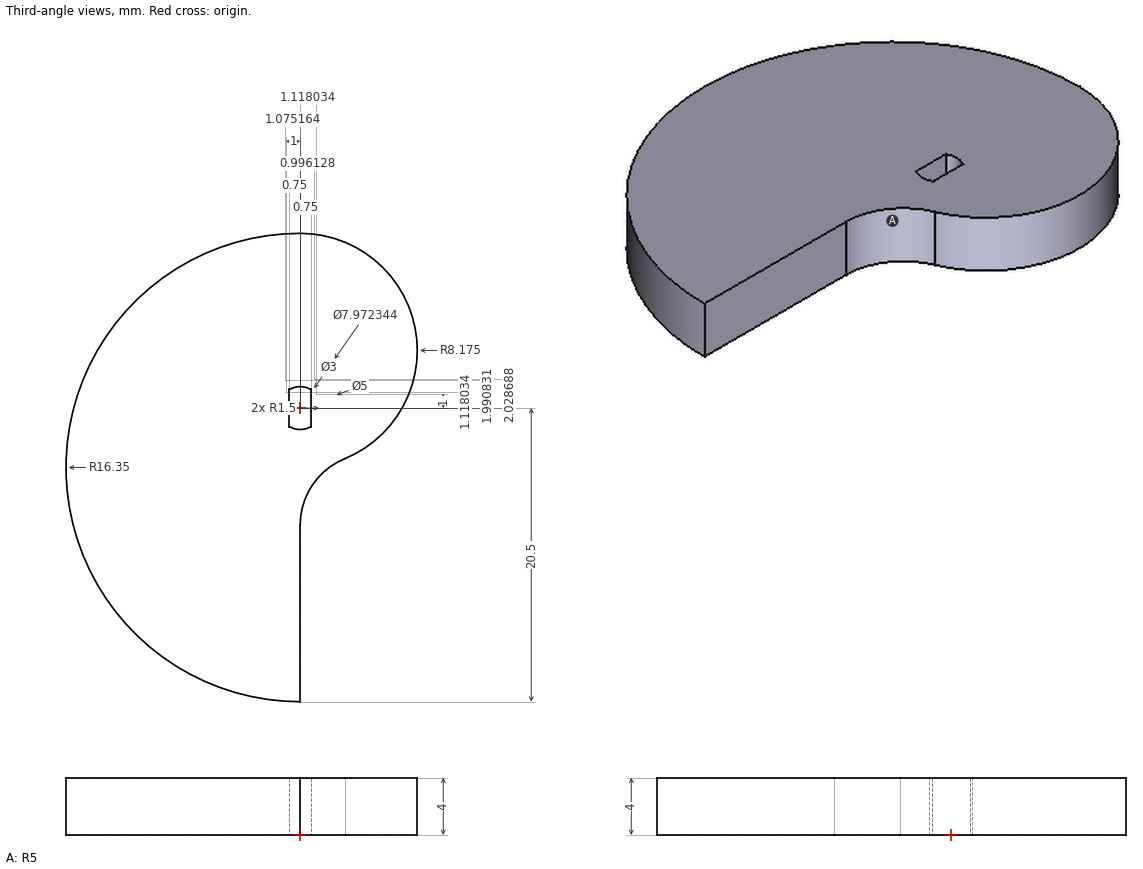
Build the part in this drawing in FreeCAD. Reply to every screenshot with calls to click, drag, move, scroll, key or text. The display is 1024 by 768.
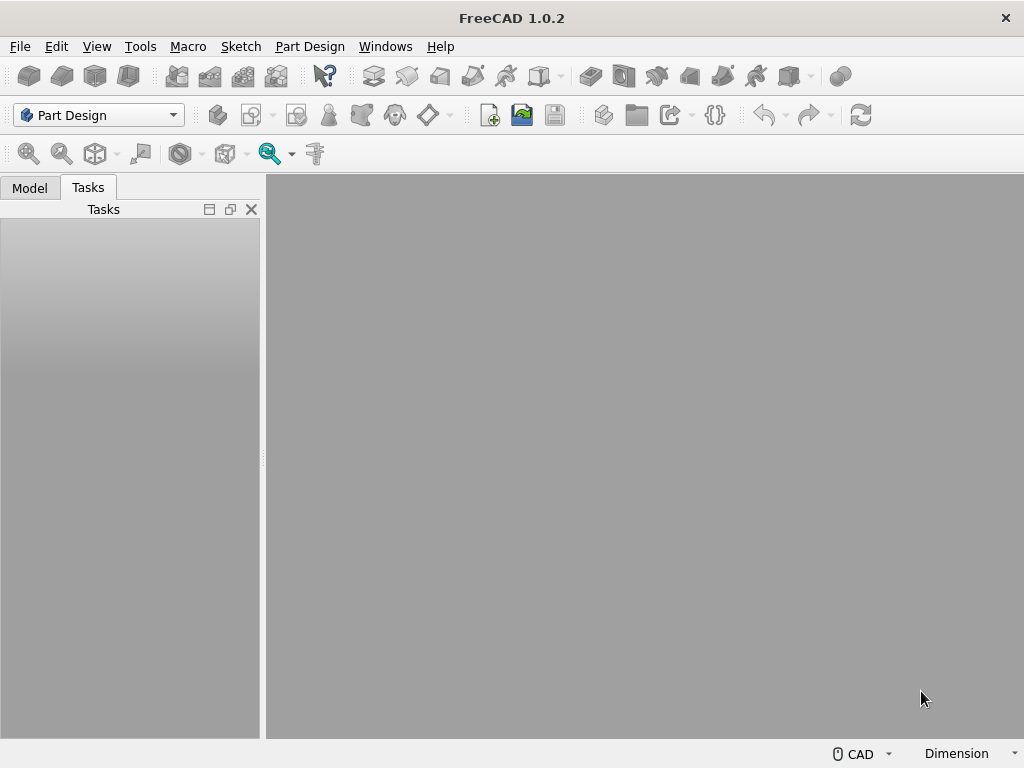
key(ctrl+n)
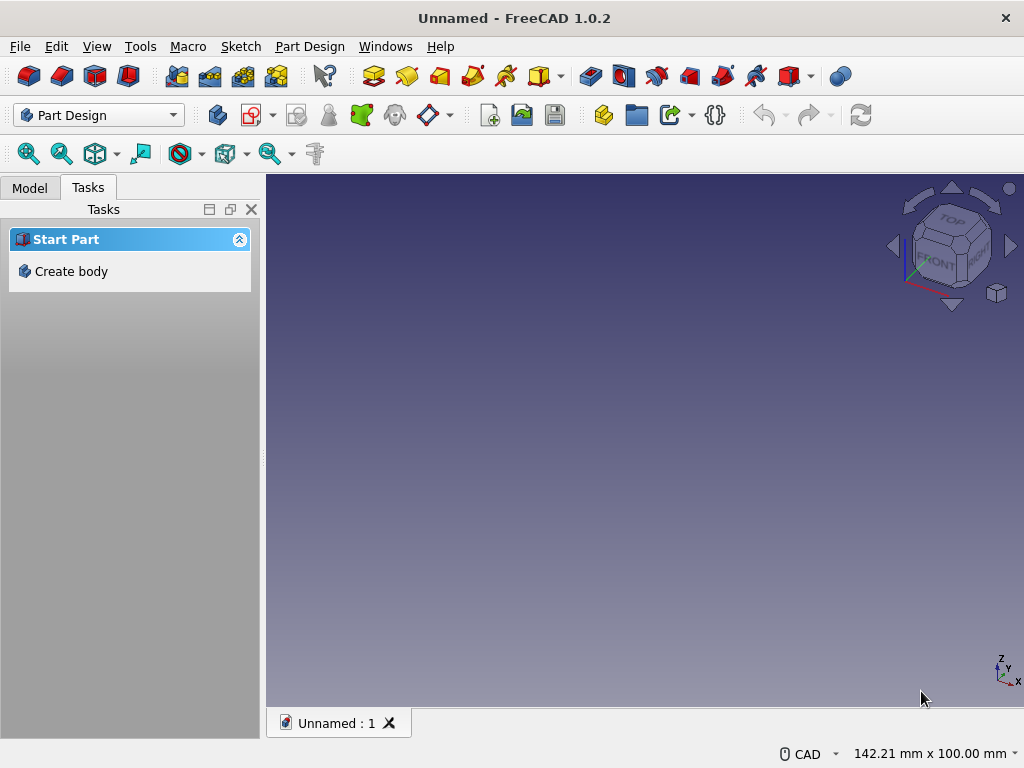
click(250, 116)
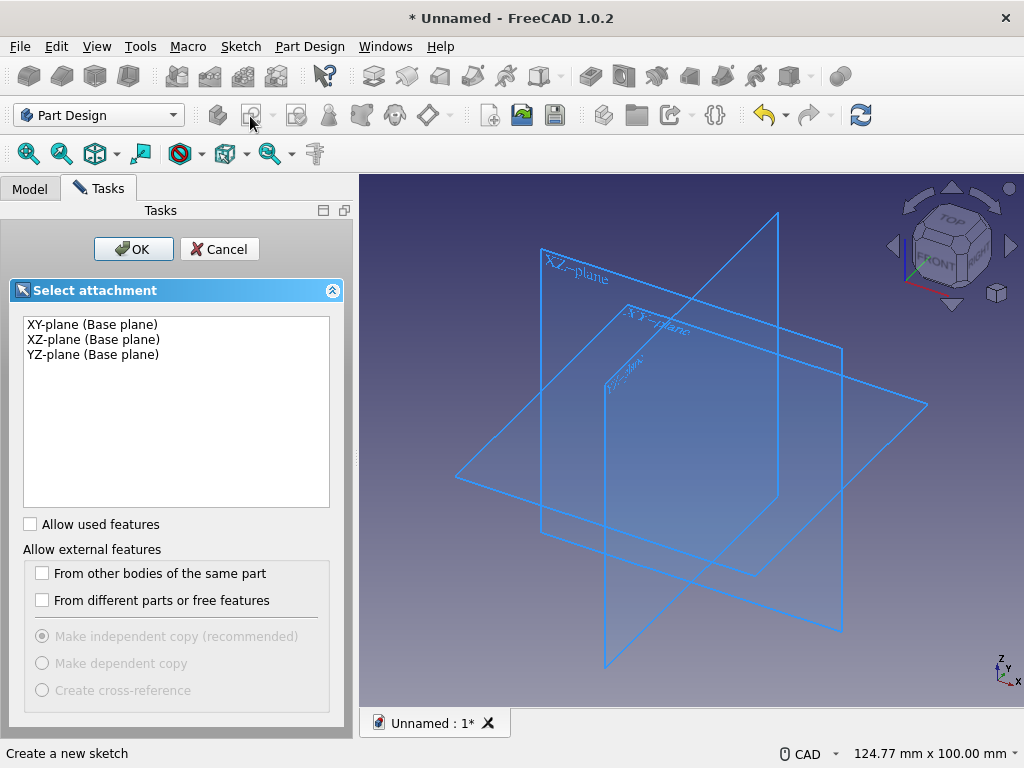
click(84, 324)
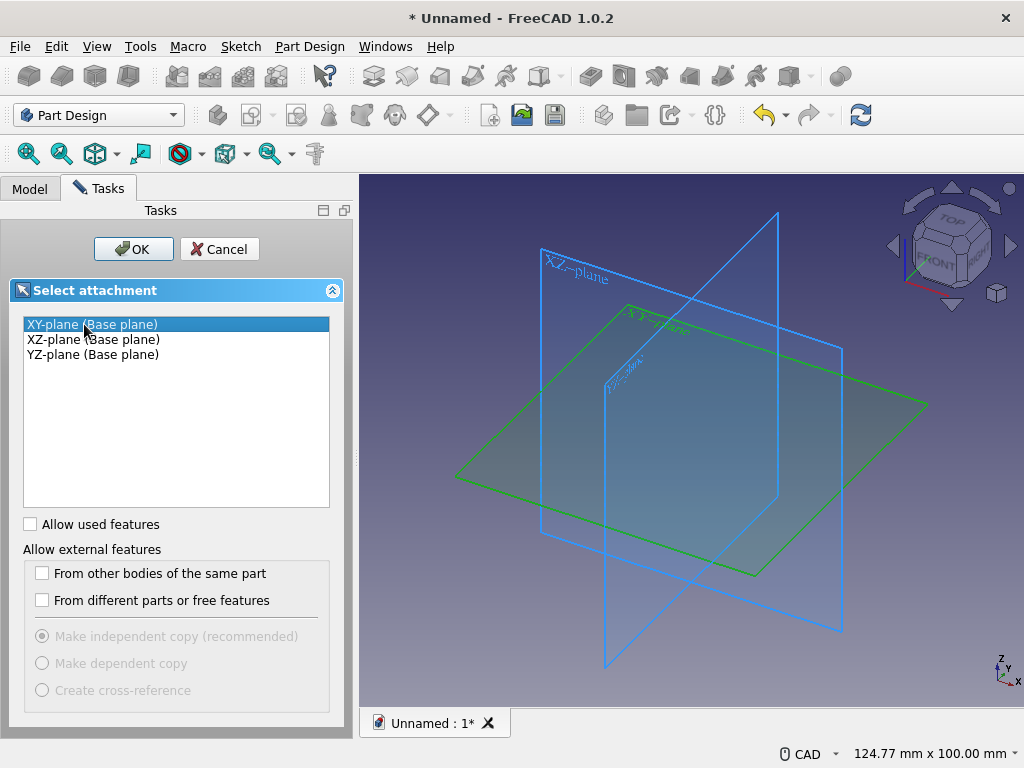
click(134, 249)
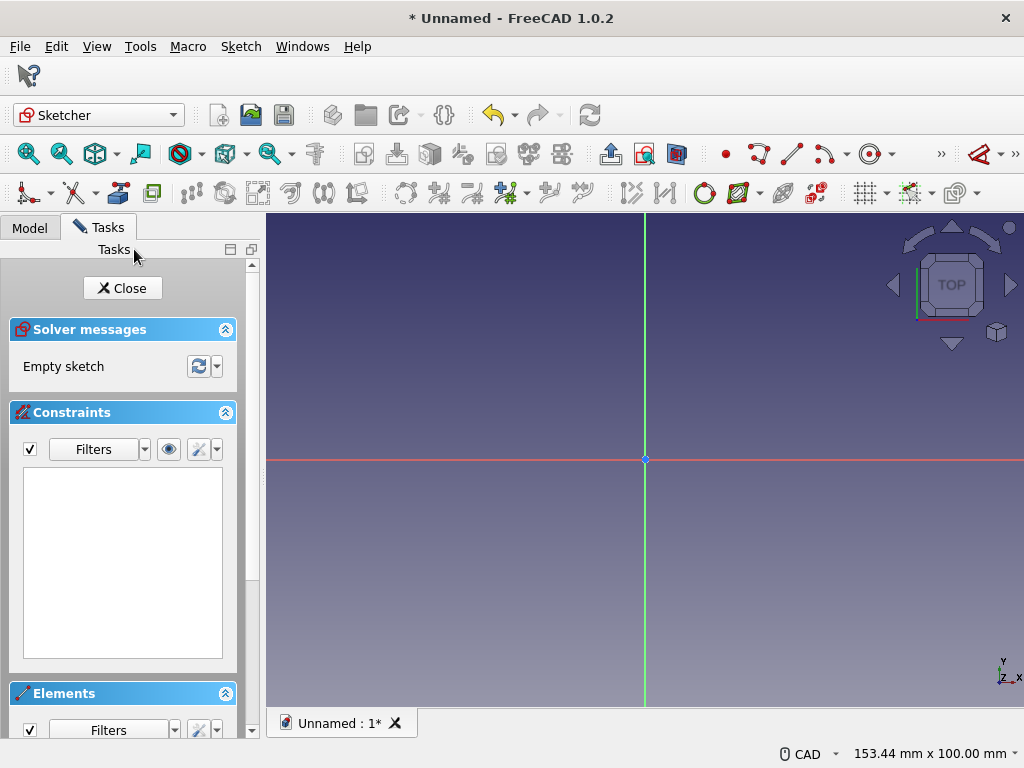
scroll(684, 505, up, 3)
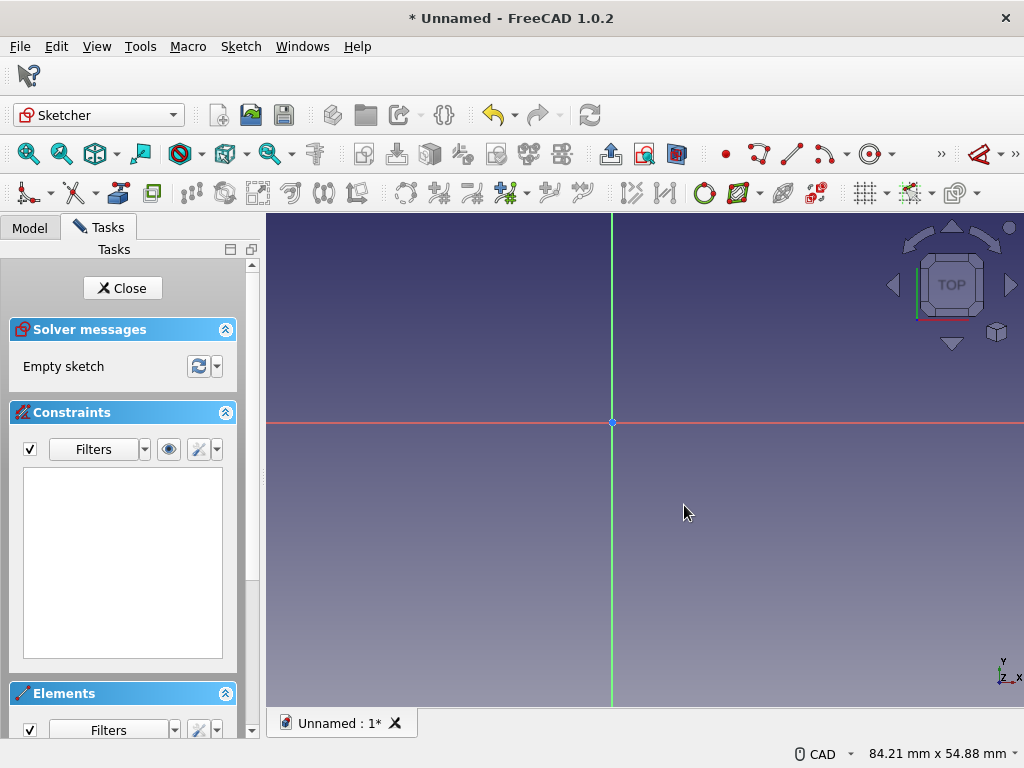
key(g)
key(l)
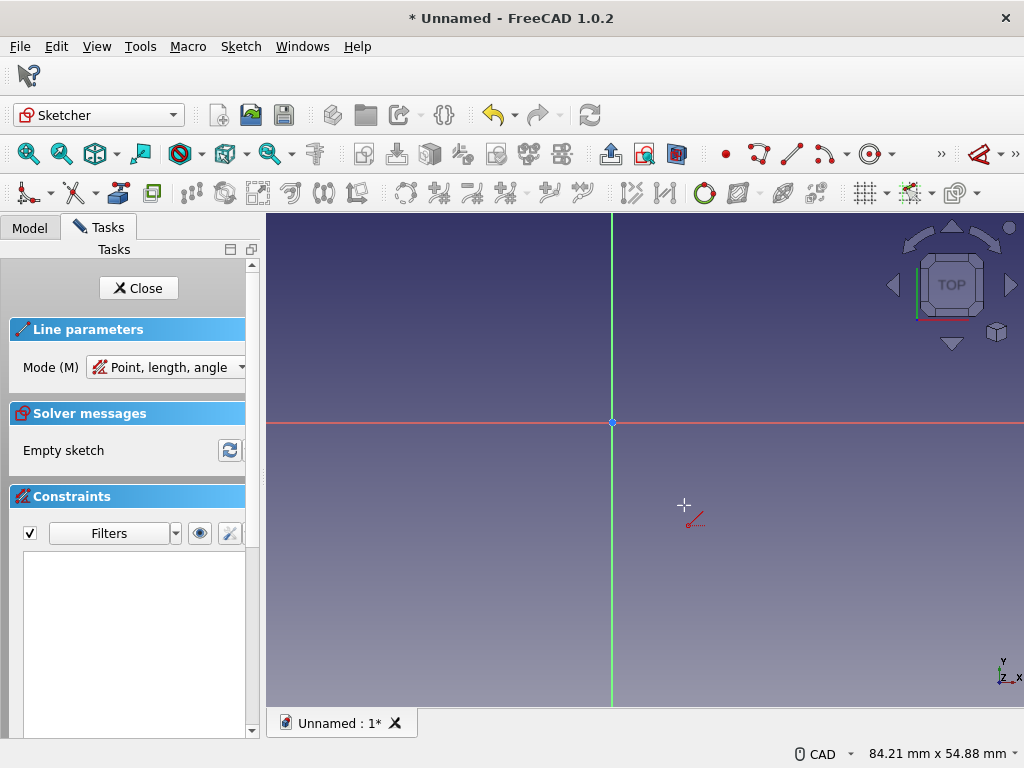
click(612, 607)
click(603, 460)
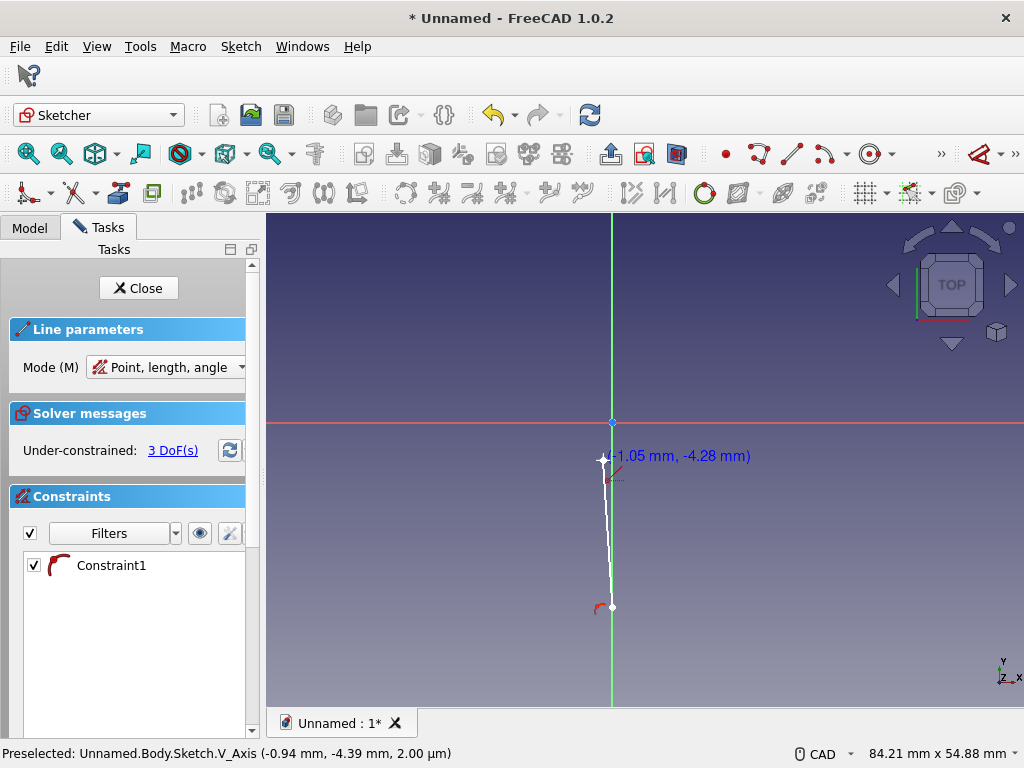
click(846, 154)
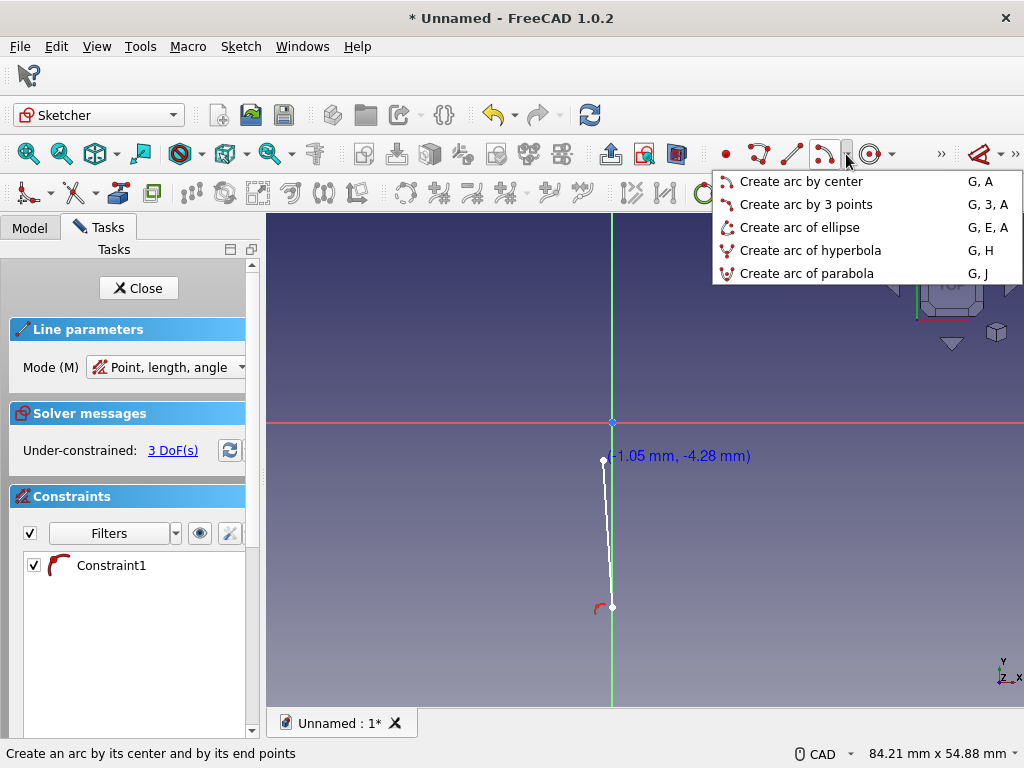
click(868, 204)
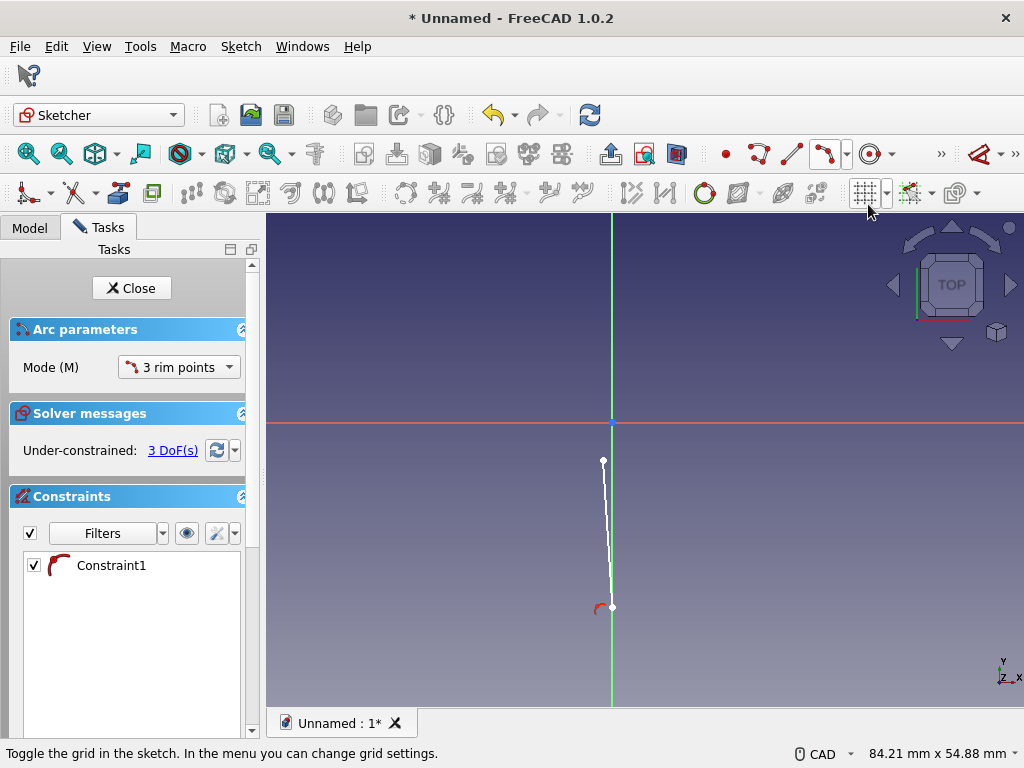
click(603, 461)
click(612, 313)
click(686, 386)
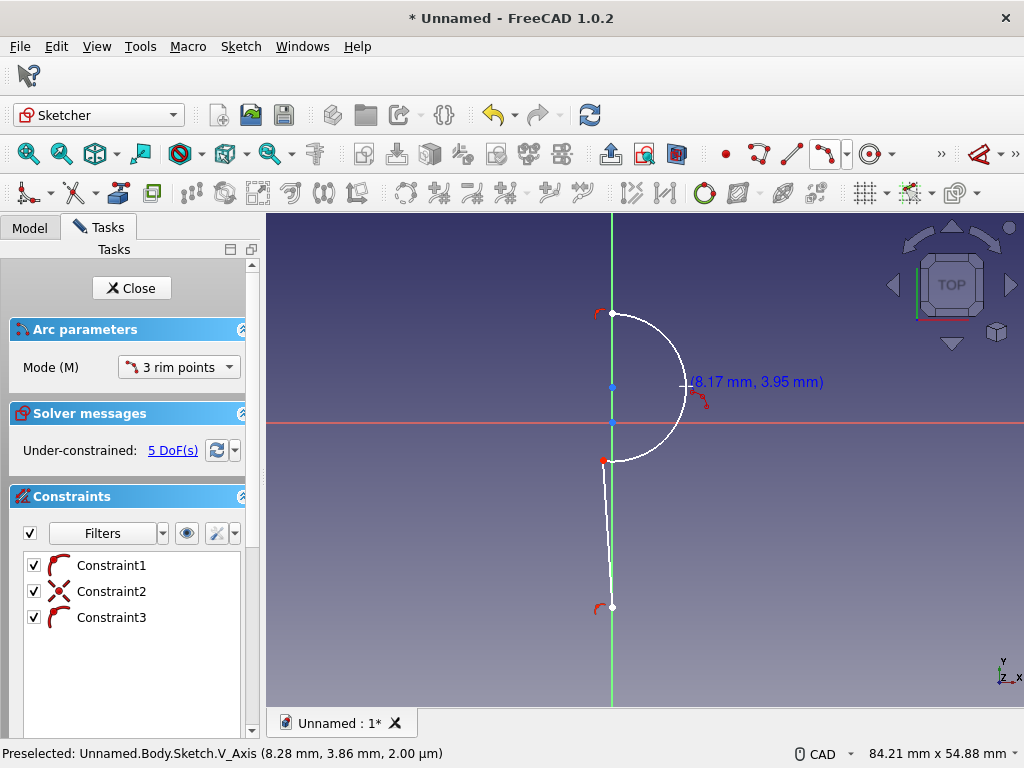
click(612, 314)
click(612, 608)
click(465, 460)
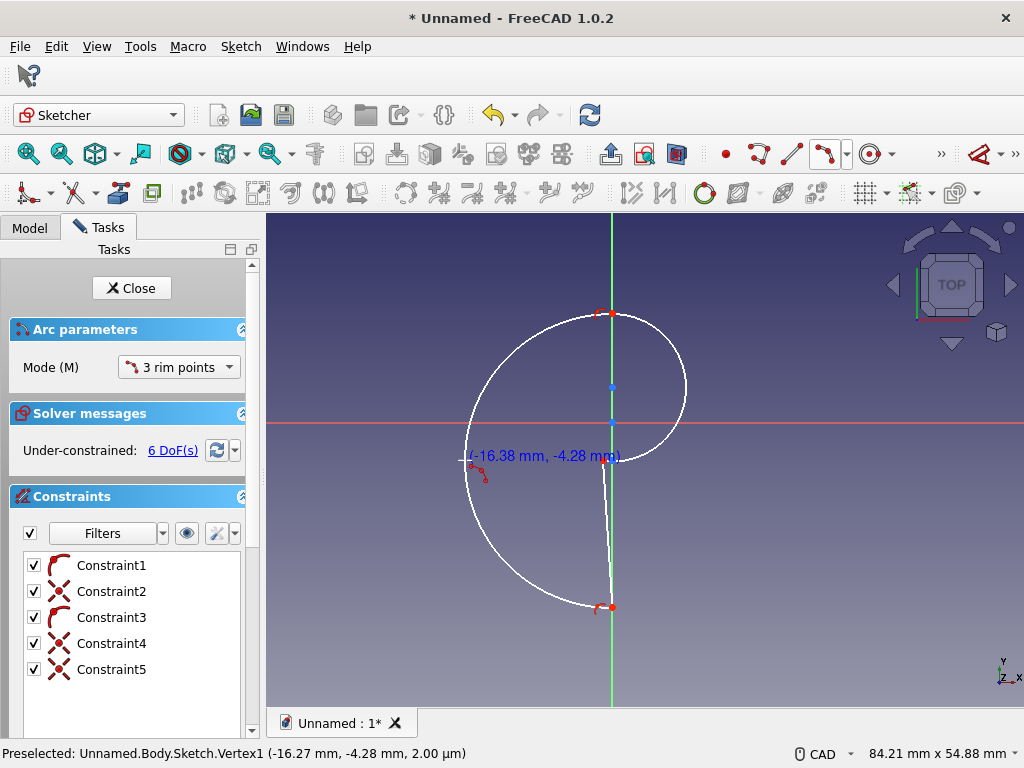
key(g)
key(c)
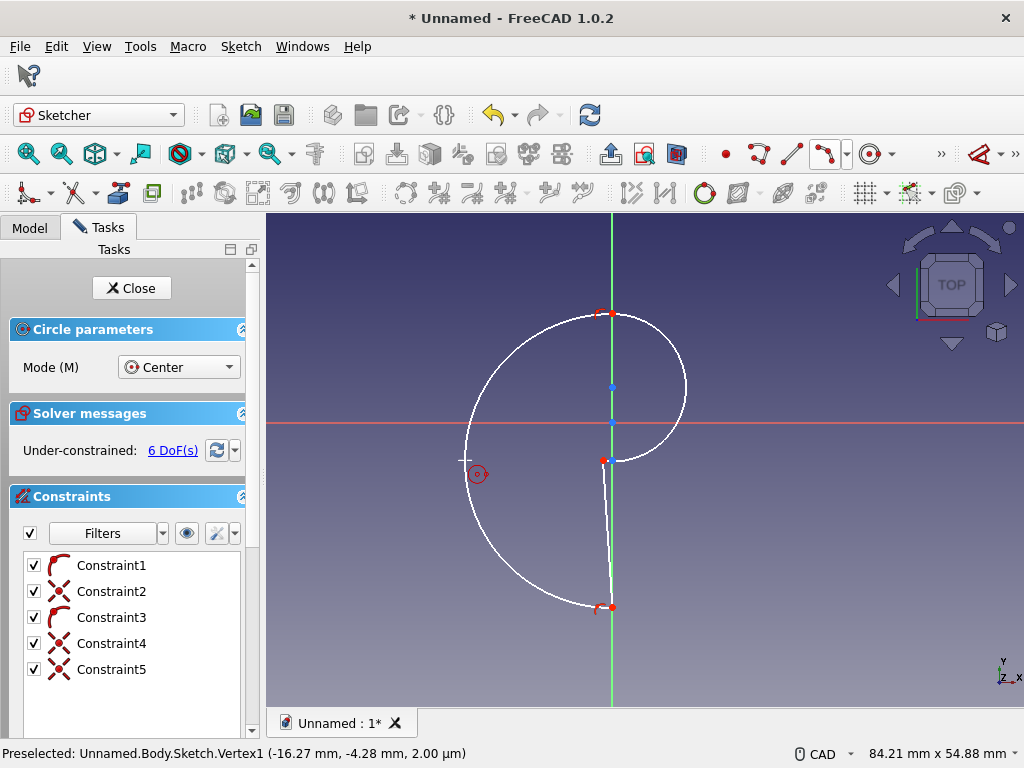
click(612, 423)
move(628, 407)